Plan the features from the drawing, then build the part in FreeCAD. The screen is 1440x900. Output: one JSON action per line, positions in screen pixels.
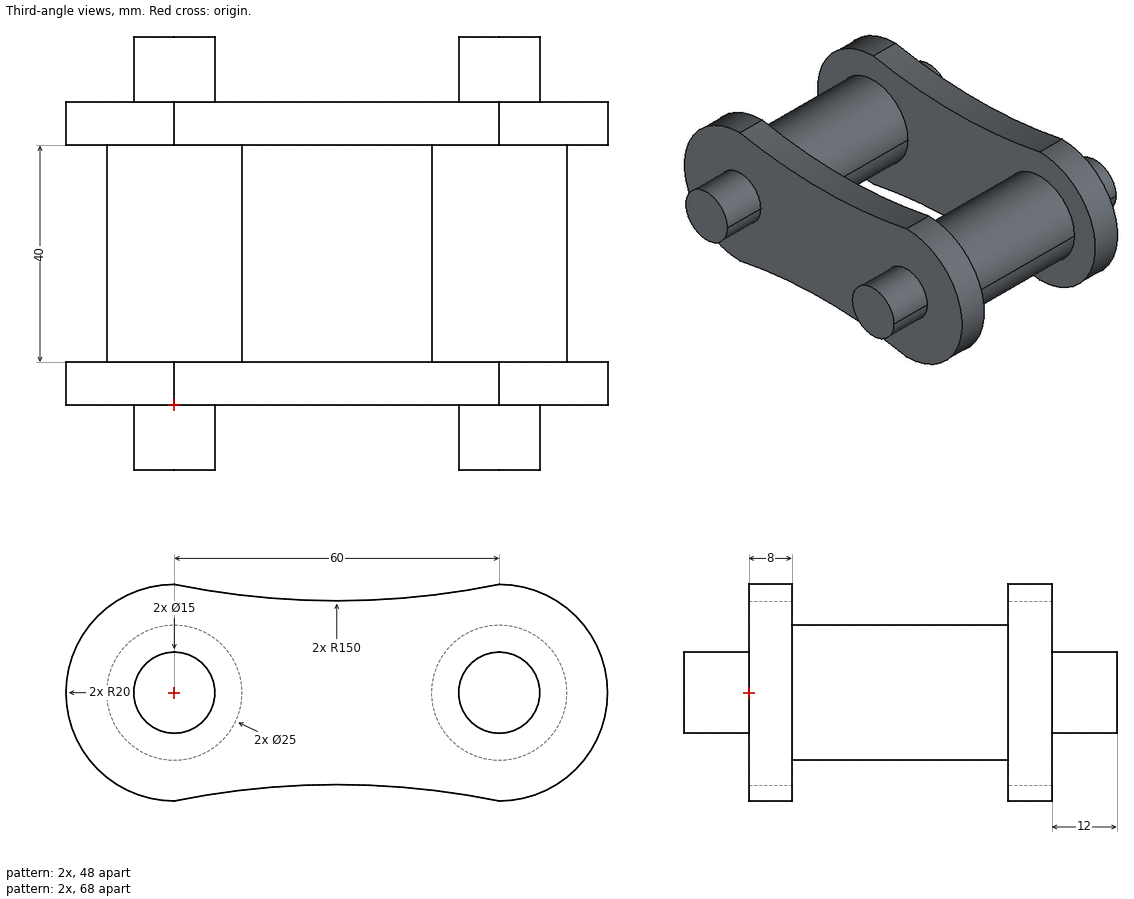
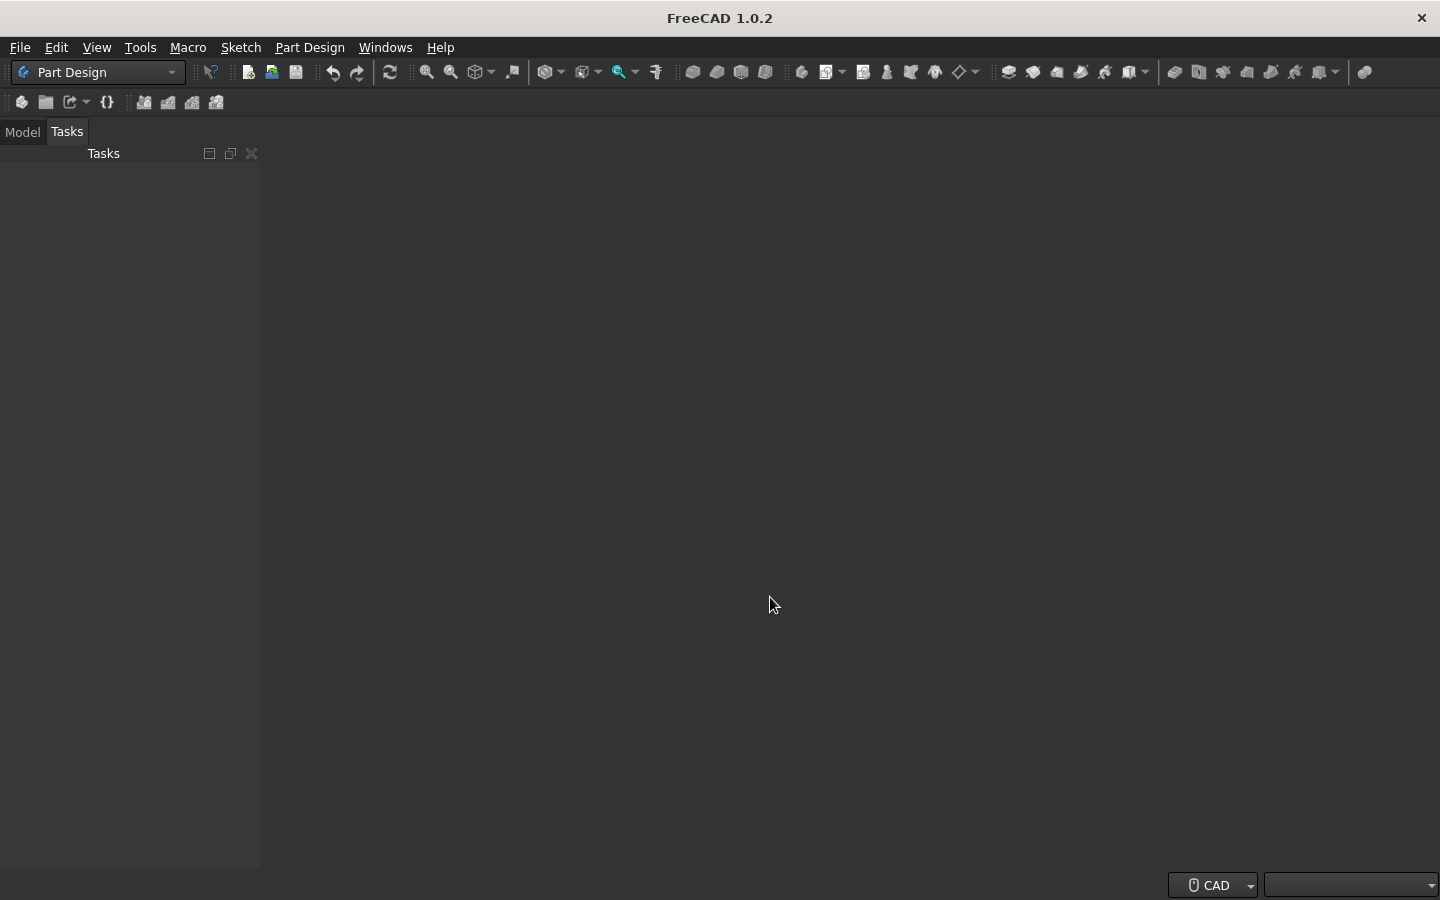
{"action": "left_click", "coordinate": [248, 72]}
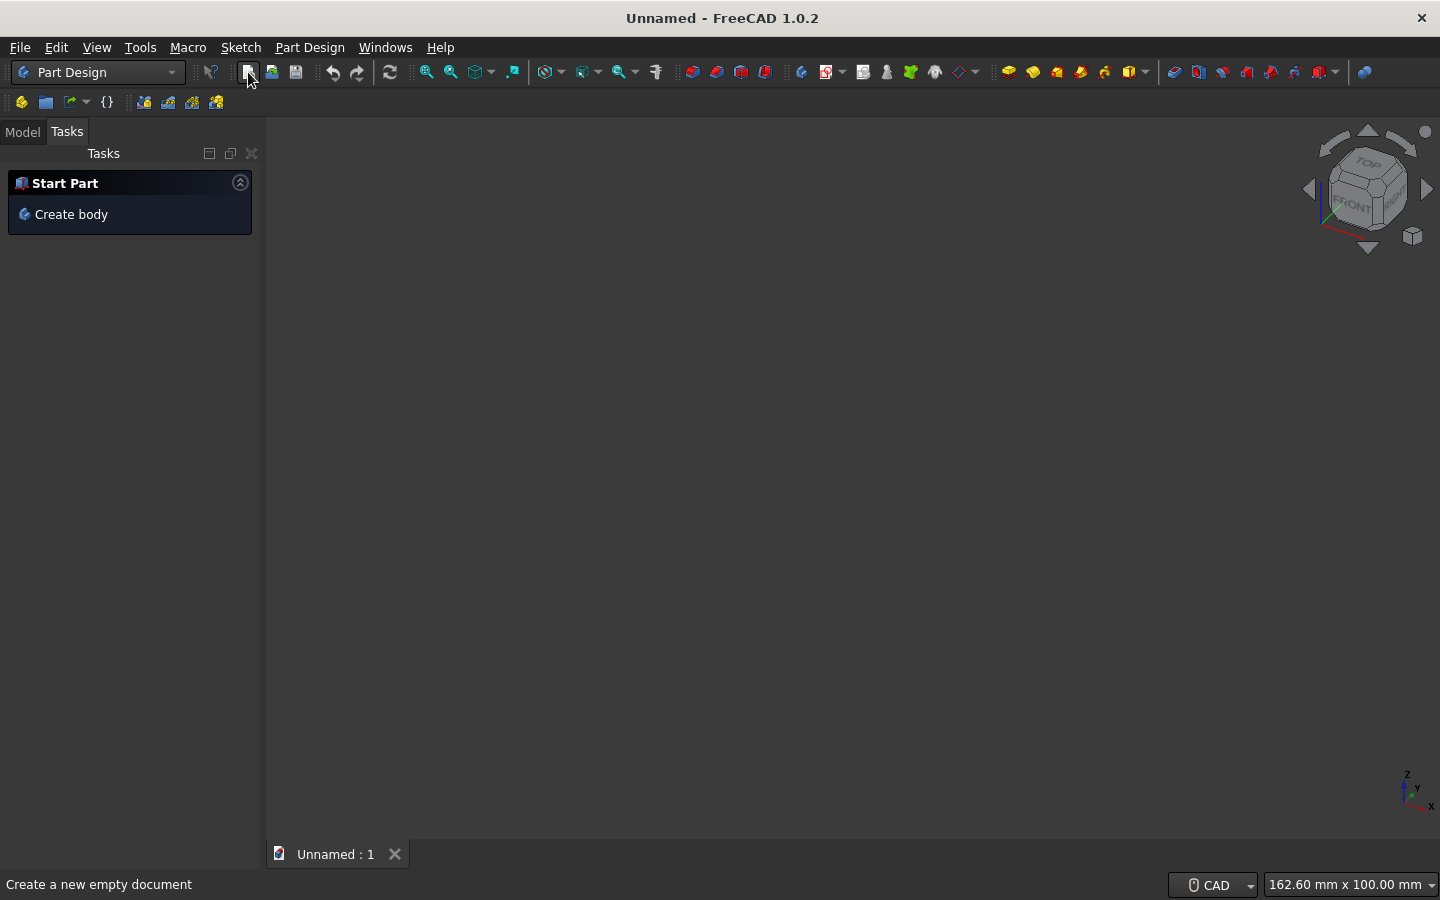
{"action": "left_click", "coordinate": [826, 72]}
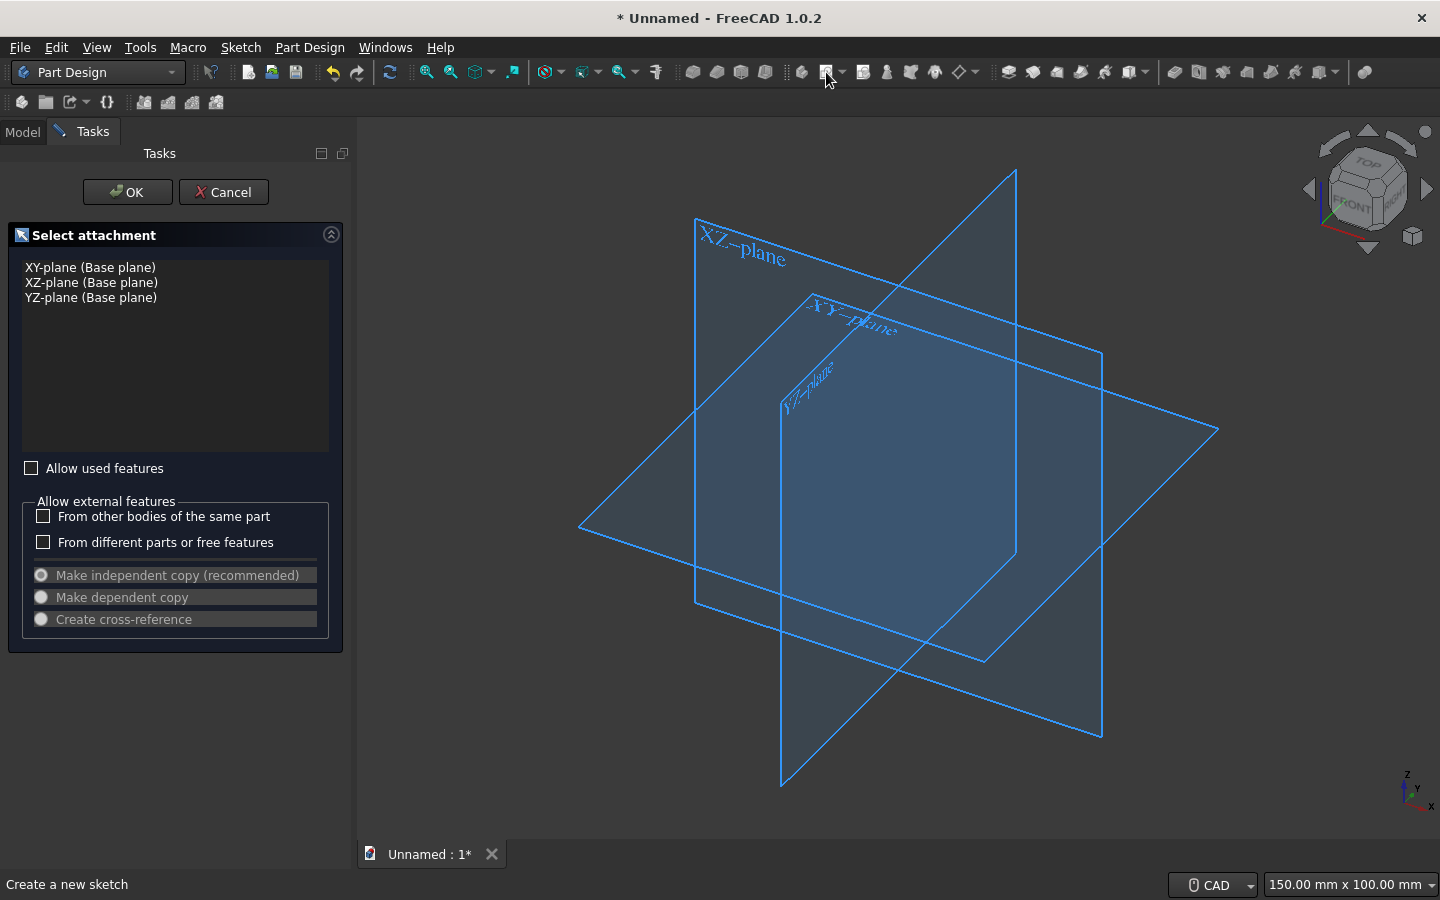
{"action": "left_click", "coordinate": [82, 282]}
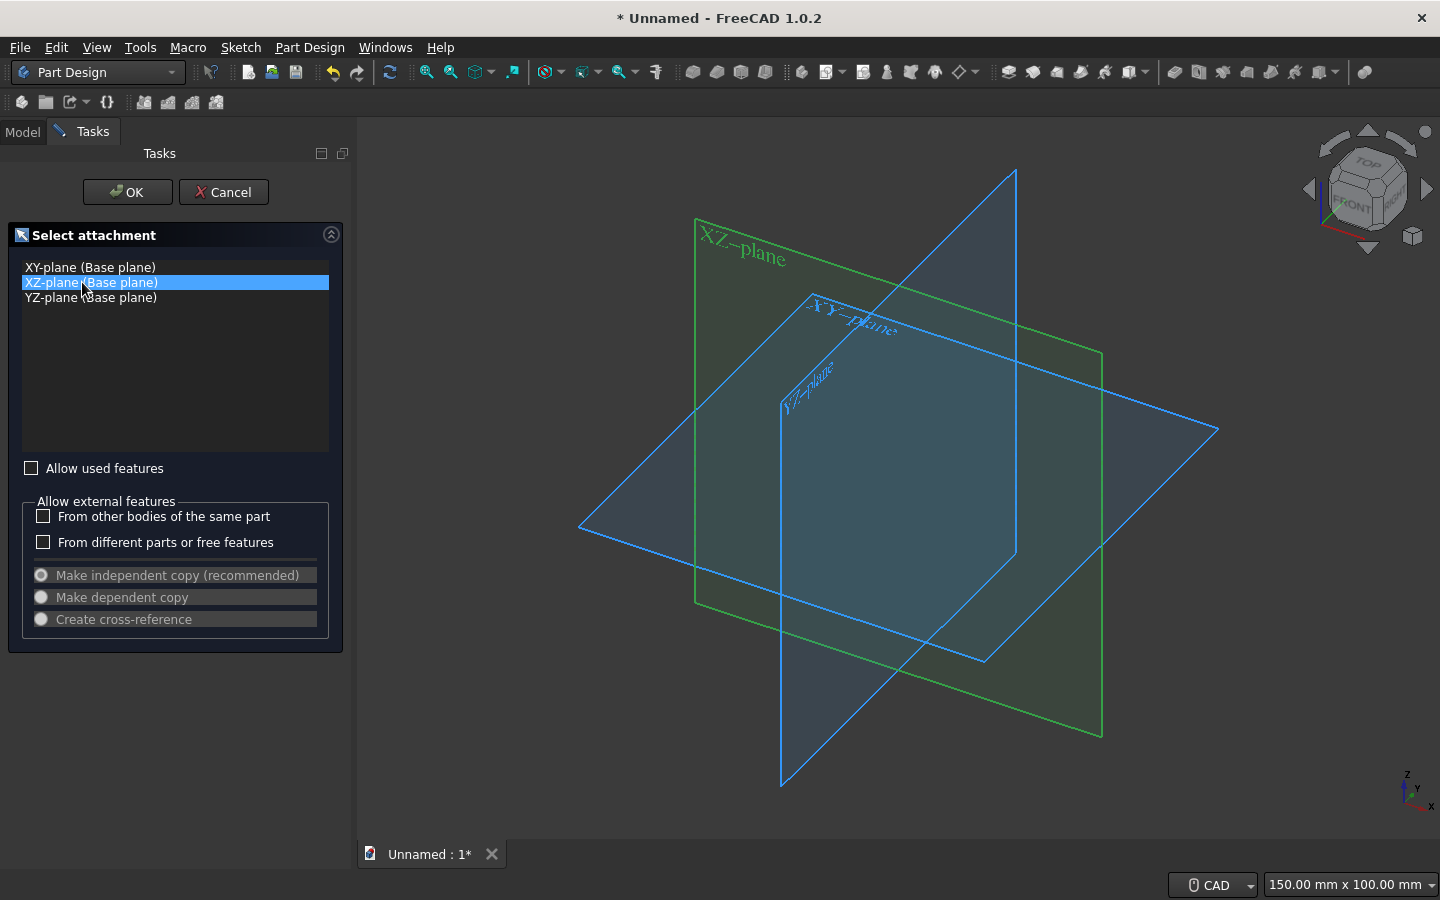
{"action": "left_click", "coordinate": [128, 192]}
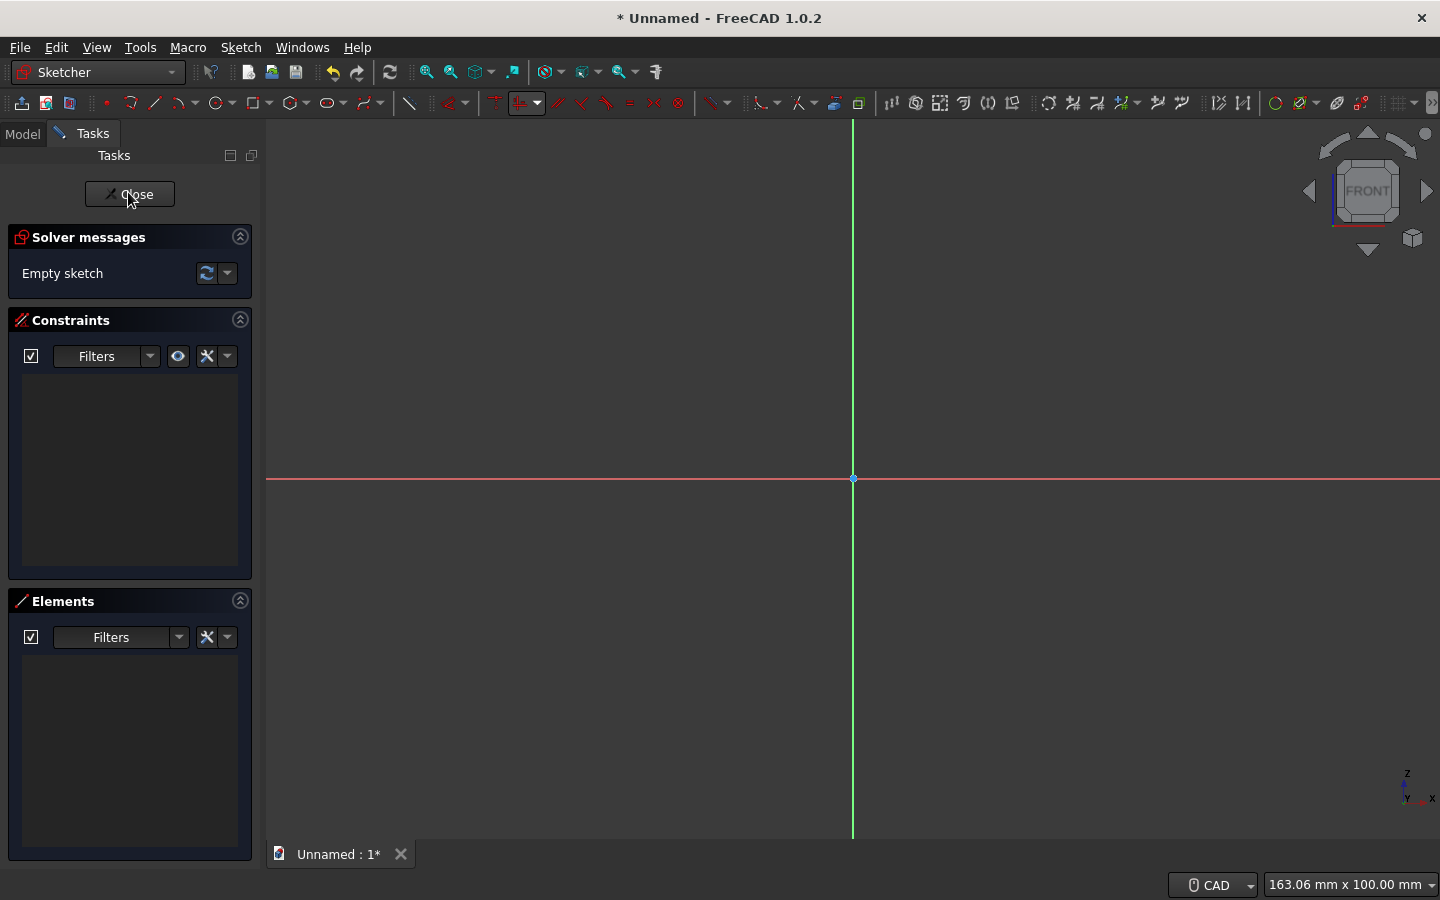
{"action": "scroll", "coordinate": [294, 479], "scroll_direction": "down", "scroll_amount": 1}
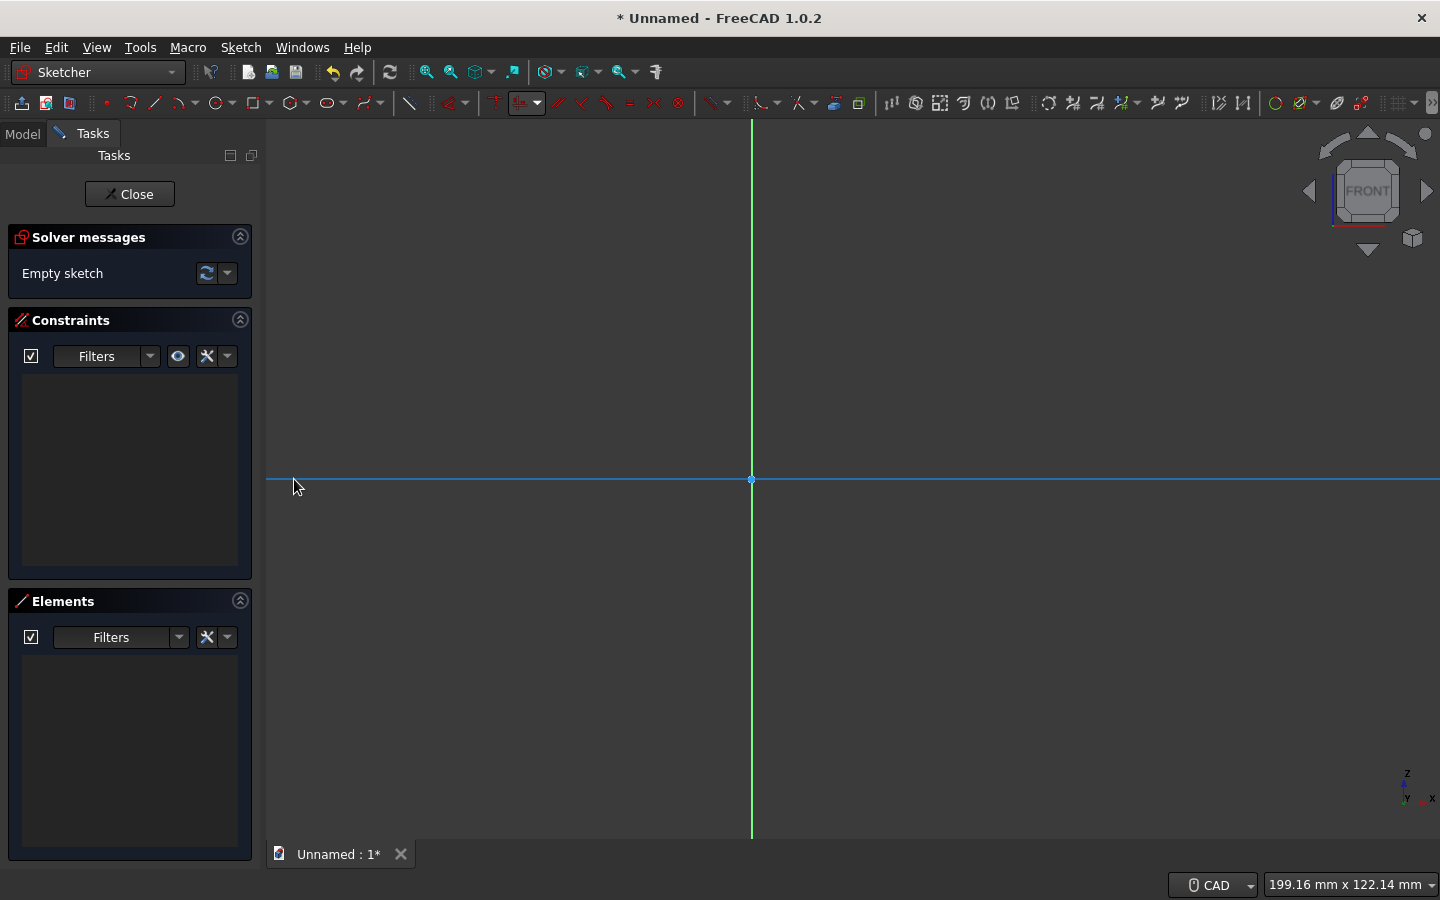
{"action": "left_click", "coordinate": [198, 104]}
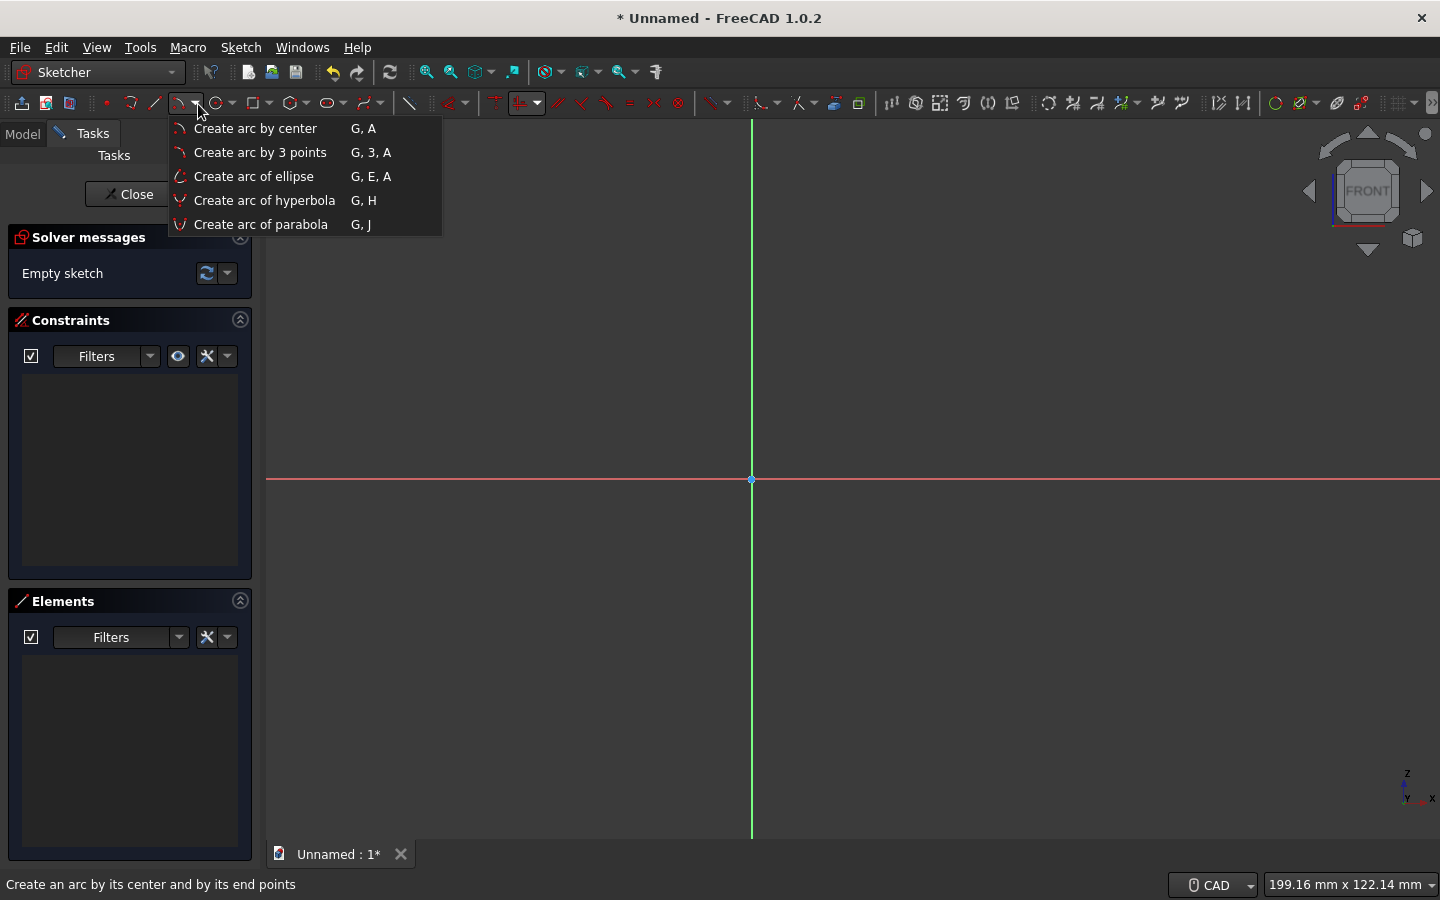
{"action": "left_click", "coordinate": [306, 152]}